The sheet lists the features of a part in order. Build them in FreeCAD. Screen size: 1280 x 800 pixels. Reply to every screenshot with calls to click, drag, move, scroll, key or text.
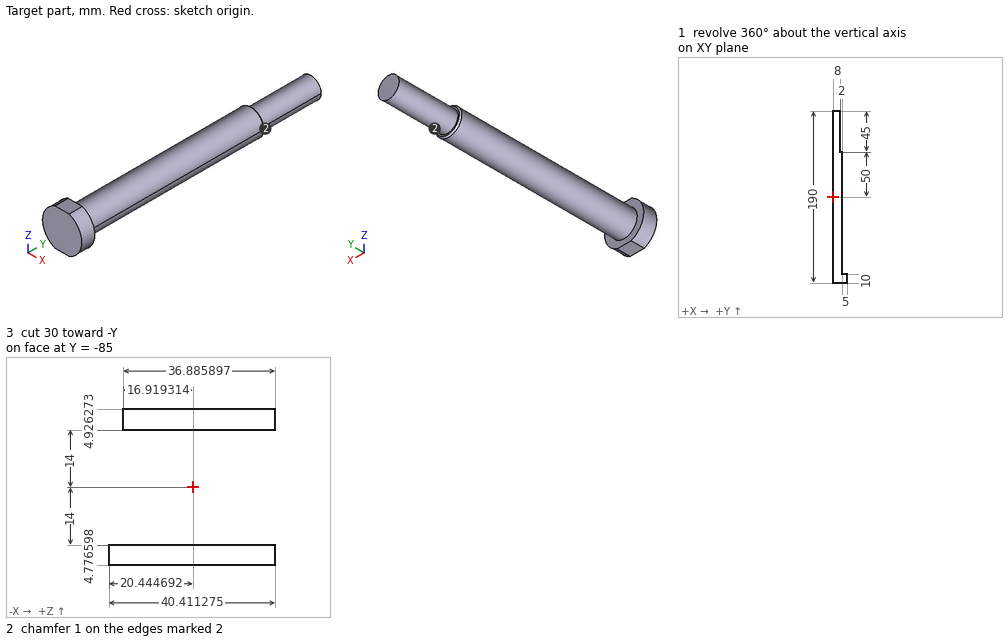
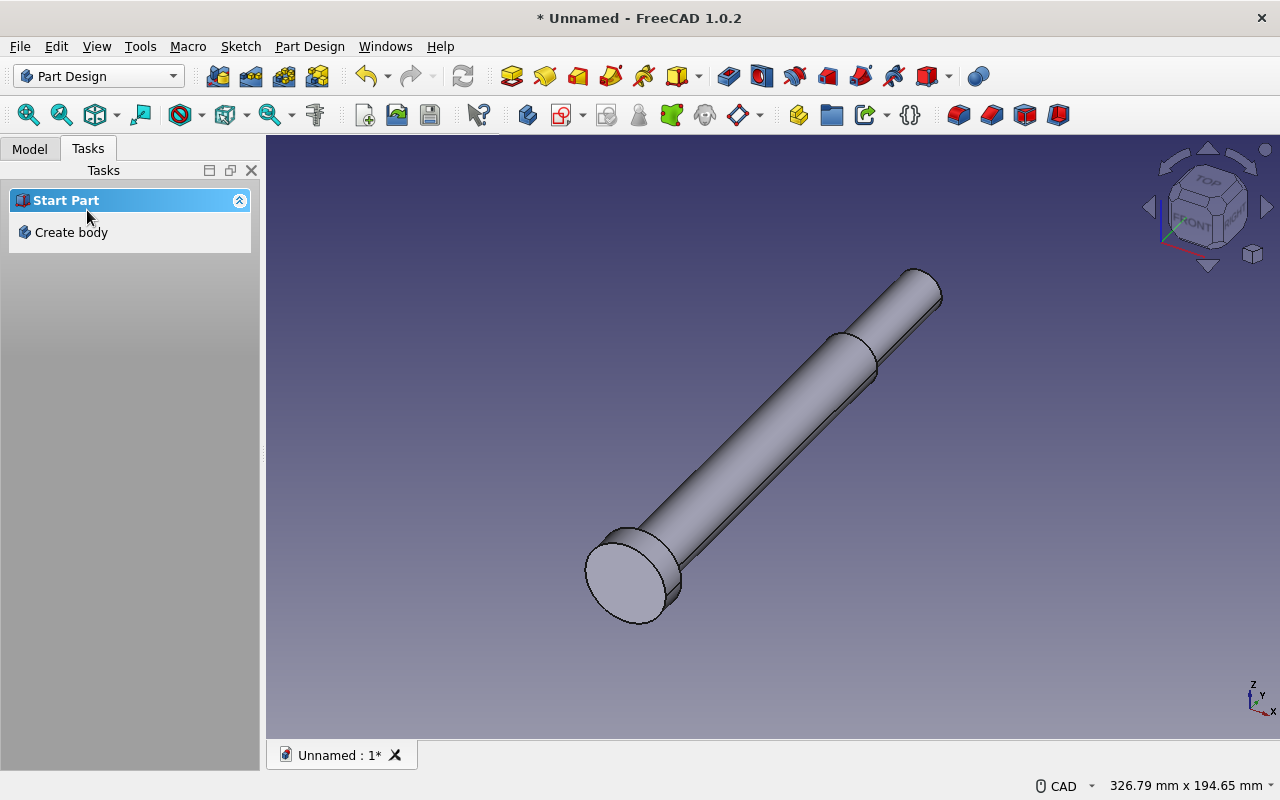
key(0)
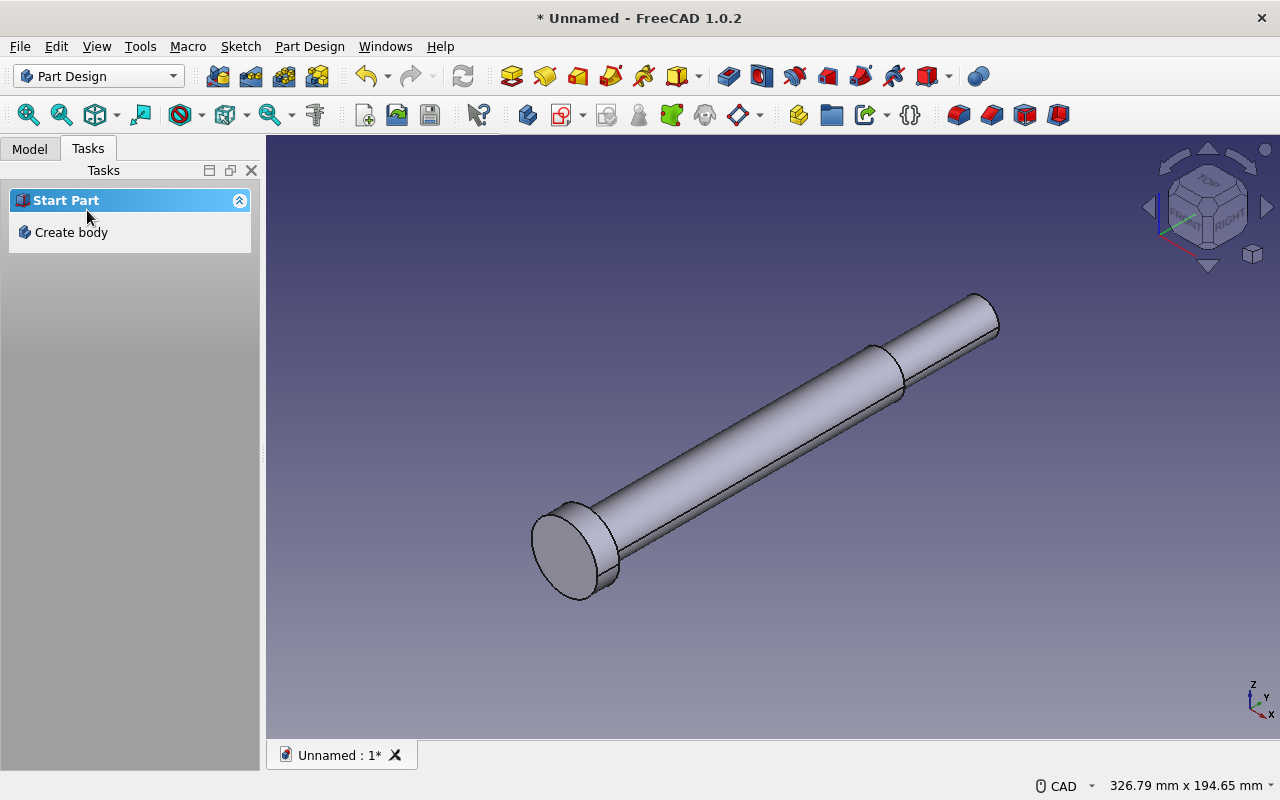
key(2)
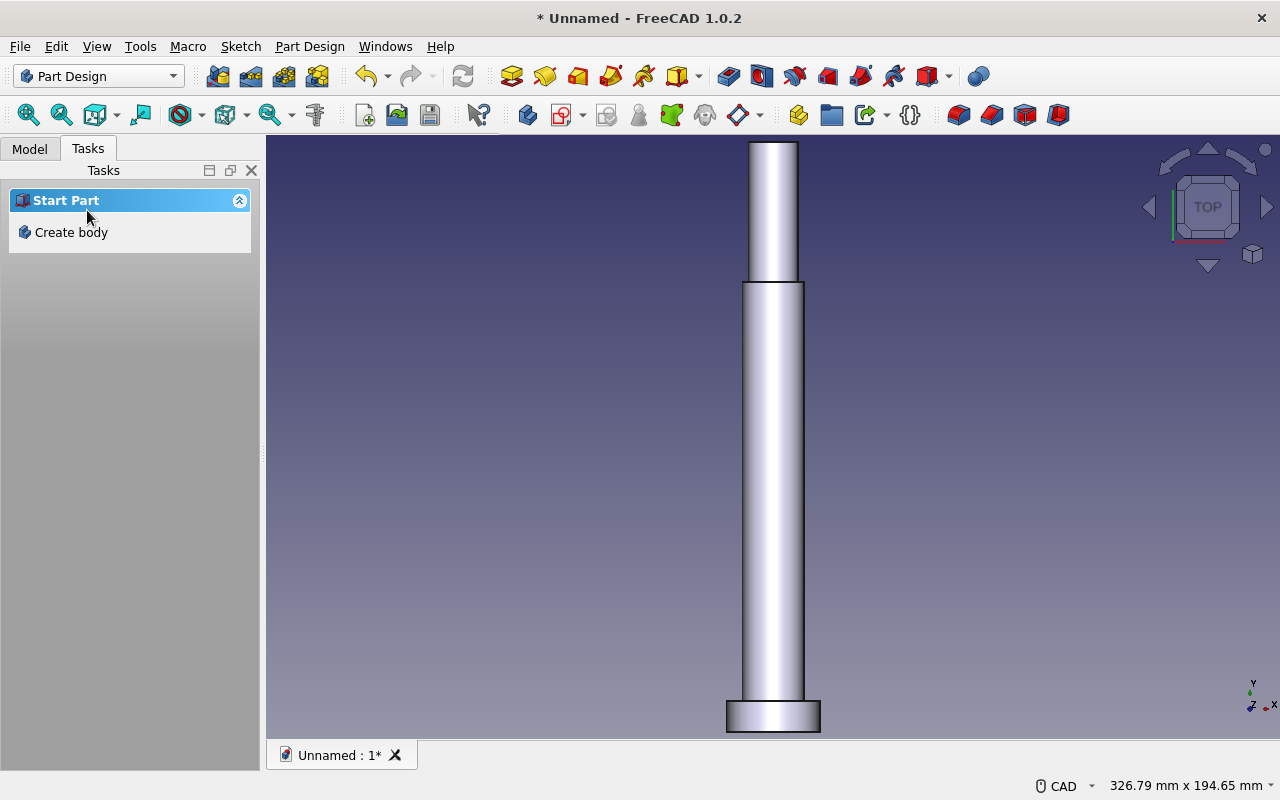
click(748, 281)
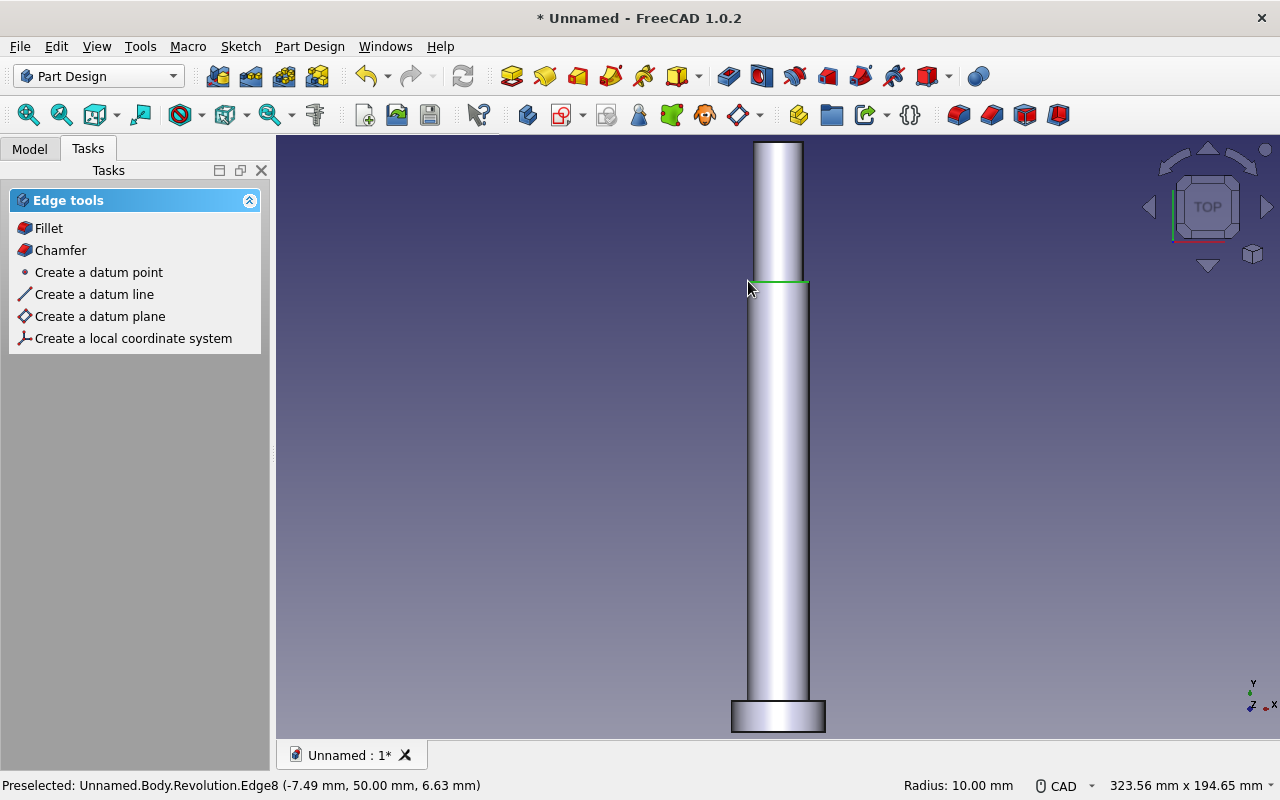
click(992, 116)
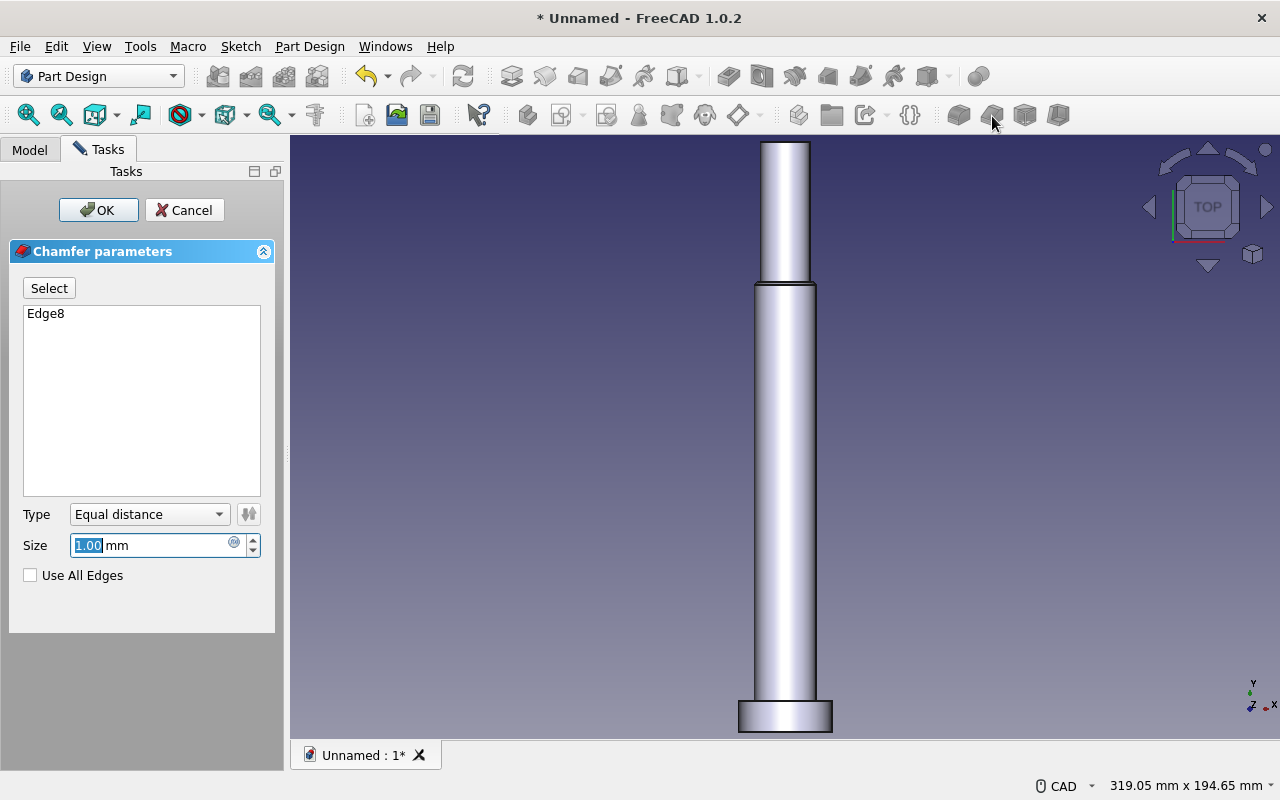
text(1)
key(Tab)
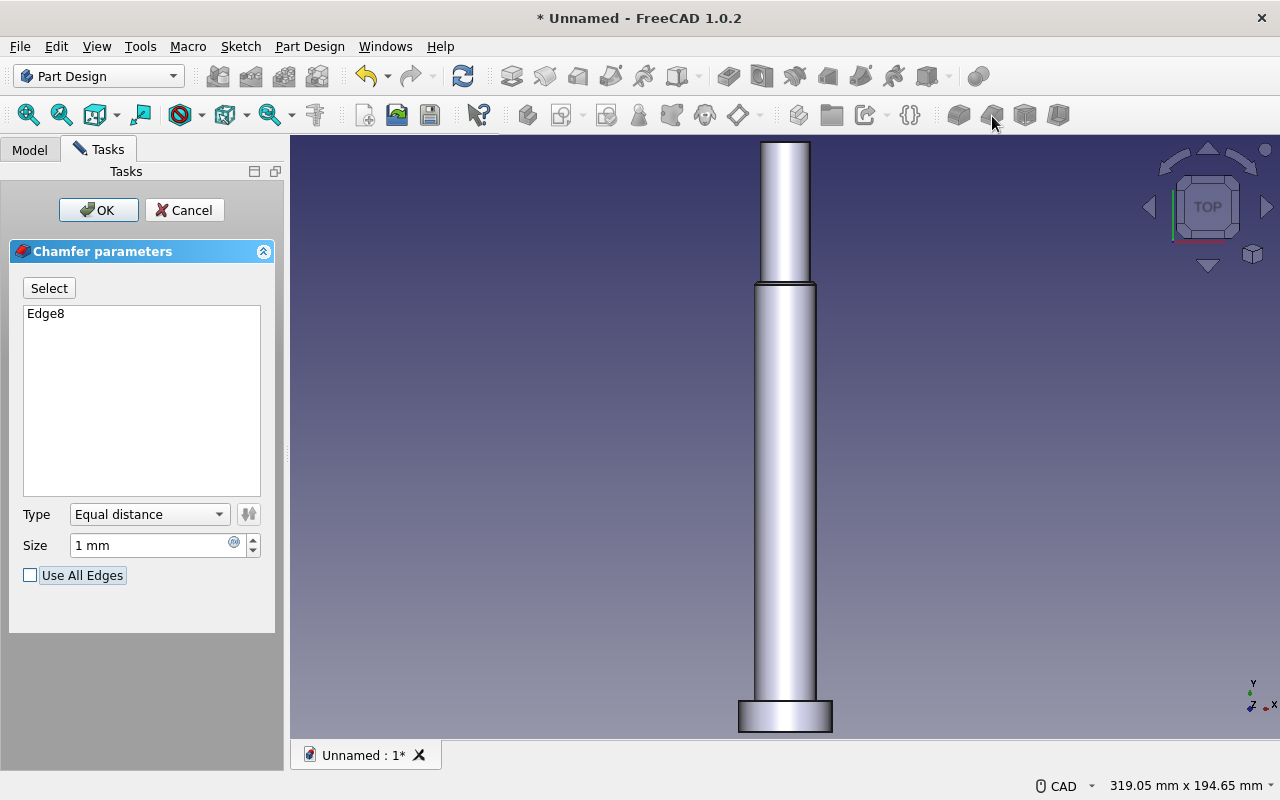
click(99, 210)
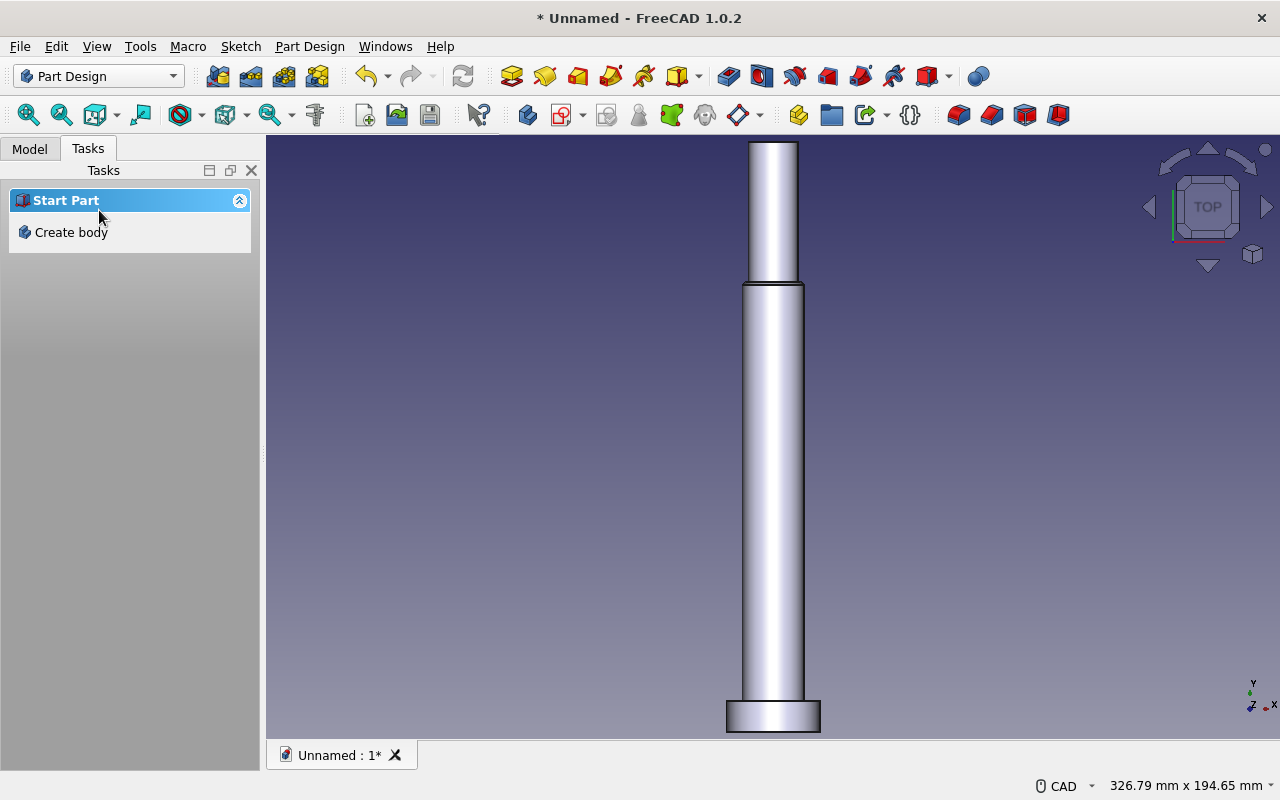
key(4)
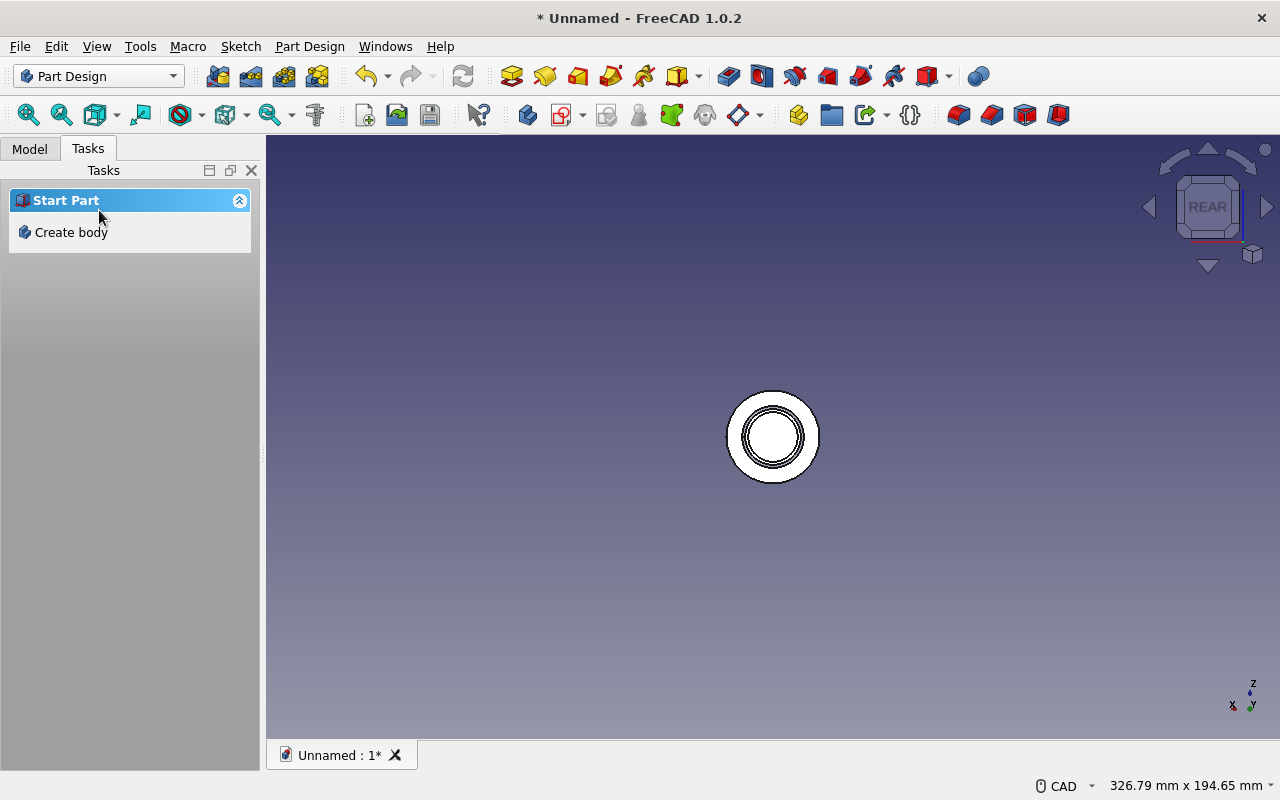
key(v)
key(f)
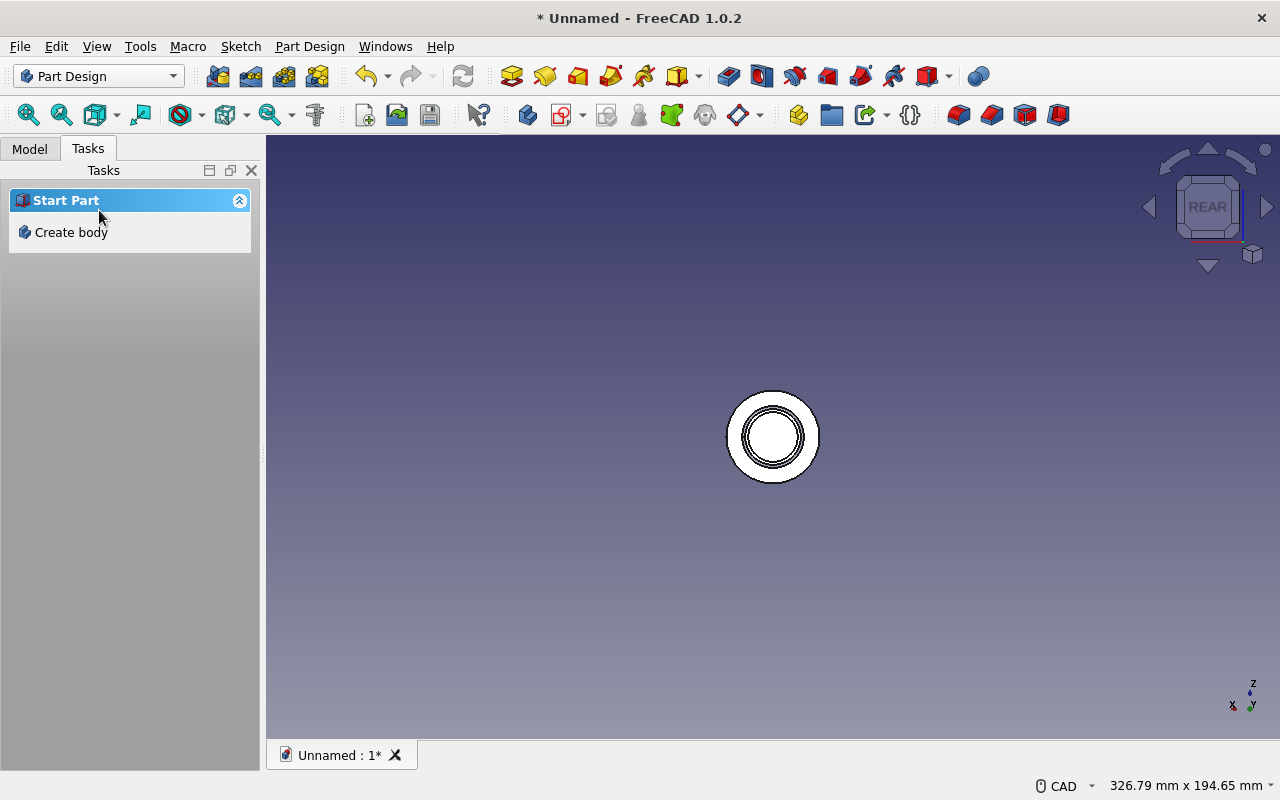
scroll(733, 436, up, 3)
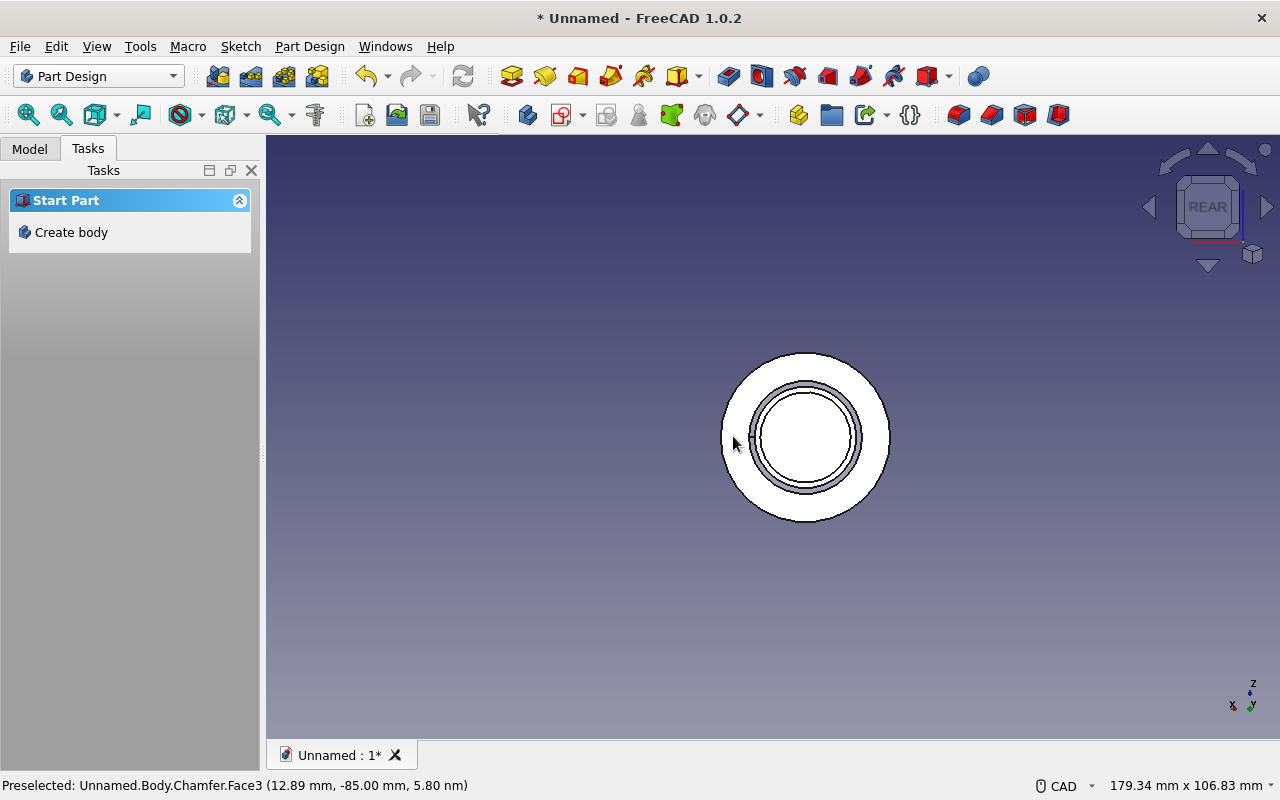
click(733, 436)